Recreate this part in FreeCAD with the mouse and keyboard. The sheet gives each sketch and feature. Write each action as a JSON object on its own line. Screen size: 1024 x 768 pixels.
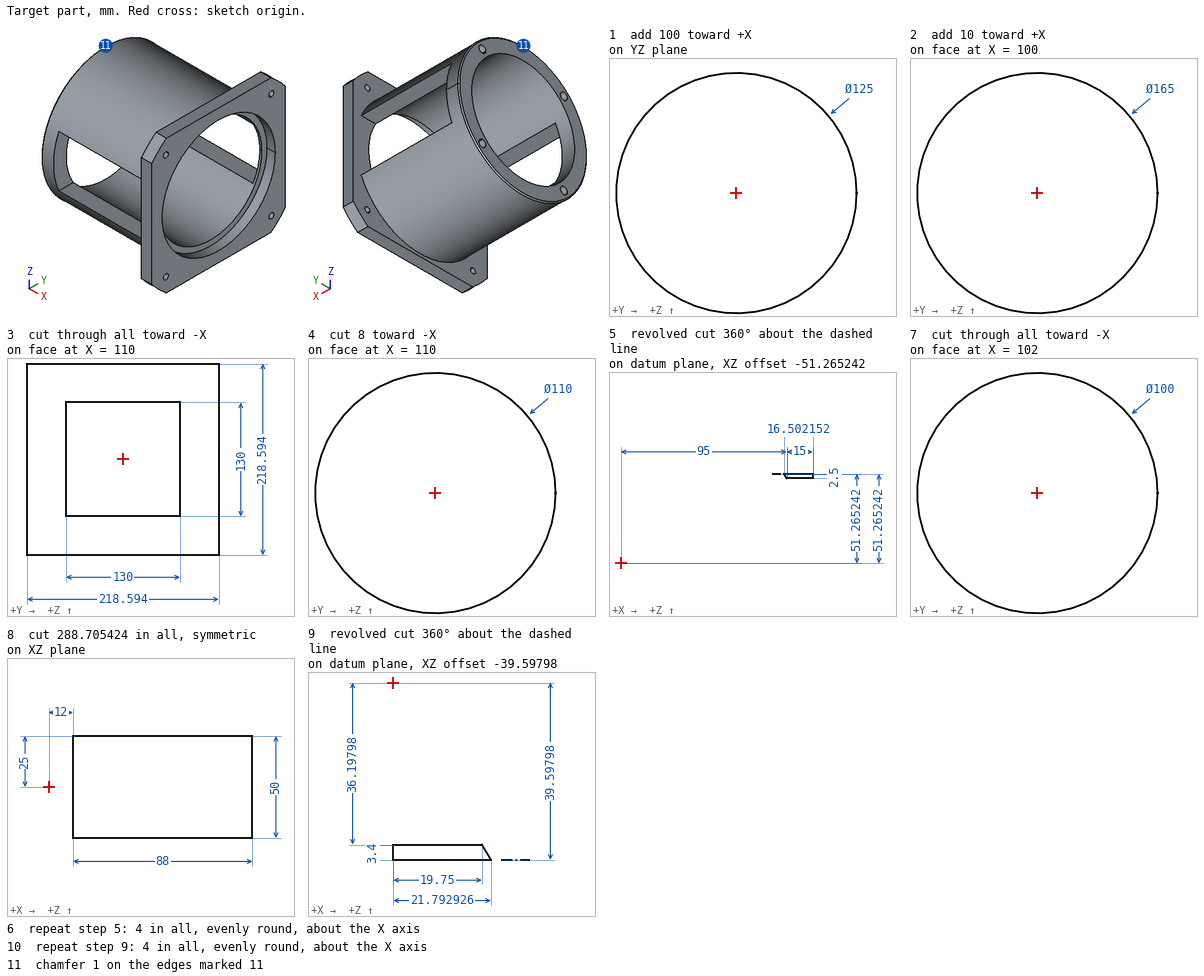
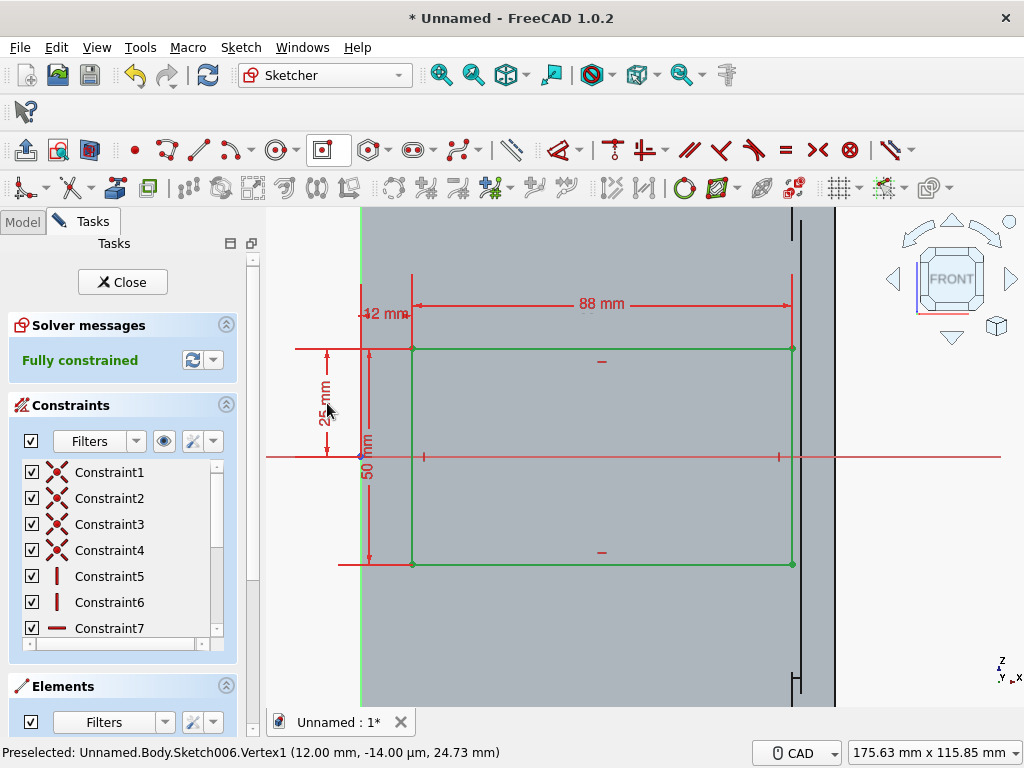
{"action": "left_click", "coordinate": [123, 282]}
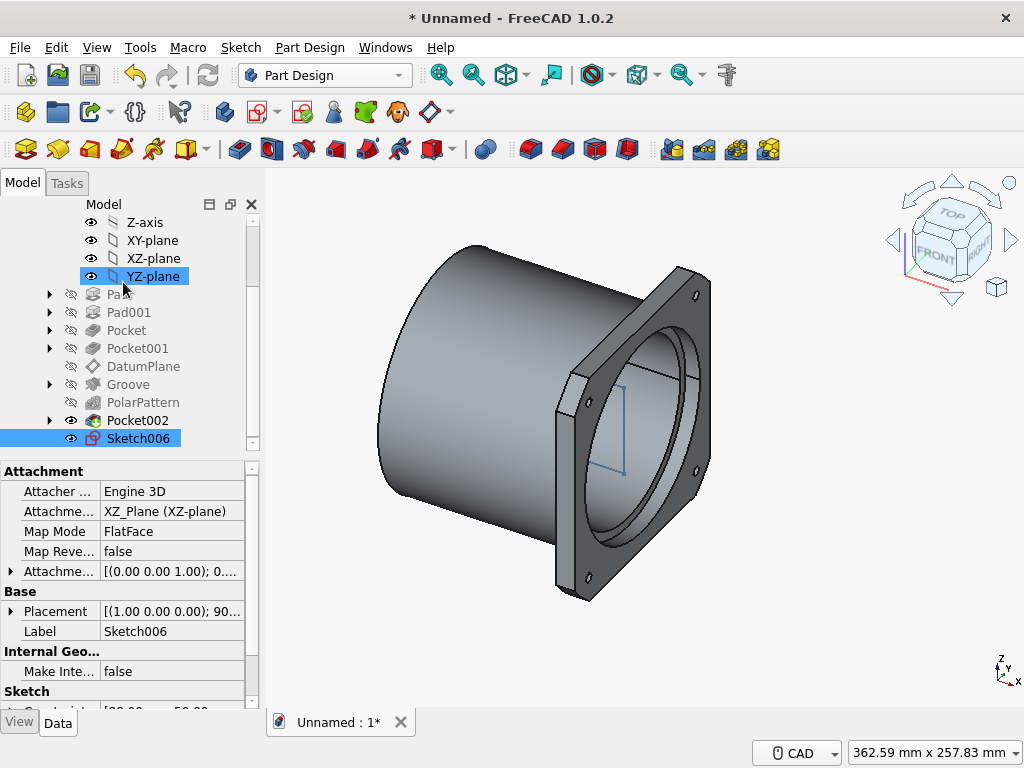
{"action": "left_click", "coordinate": [240, 150]}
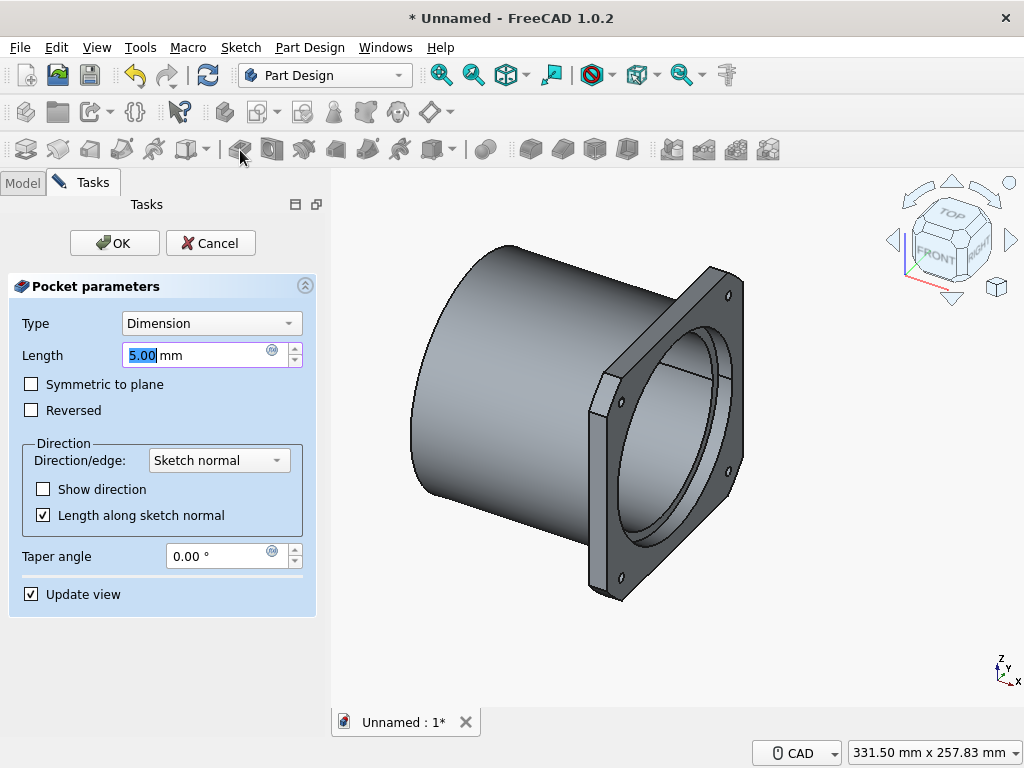
{"action": "type", "text": "288.705424"}
{"action": "key", "text": "Tab"}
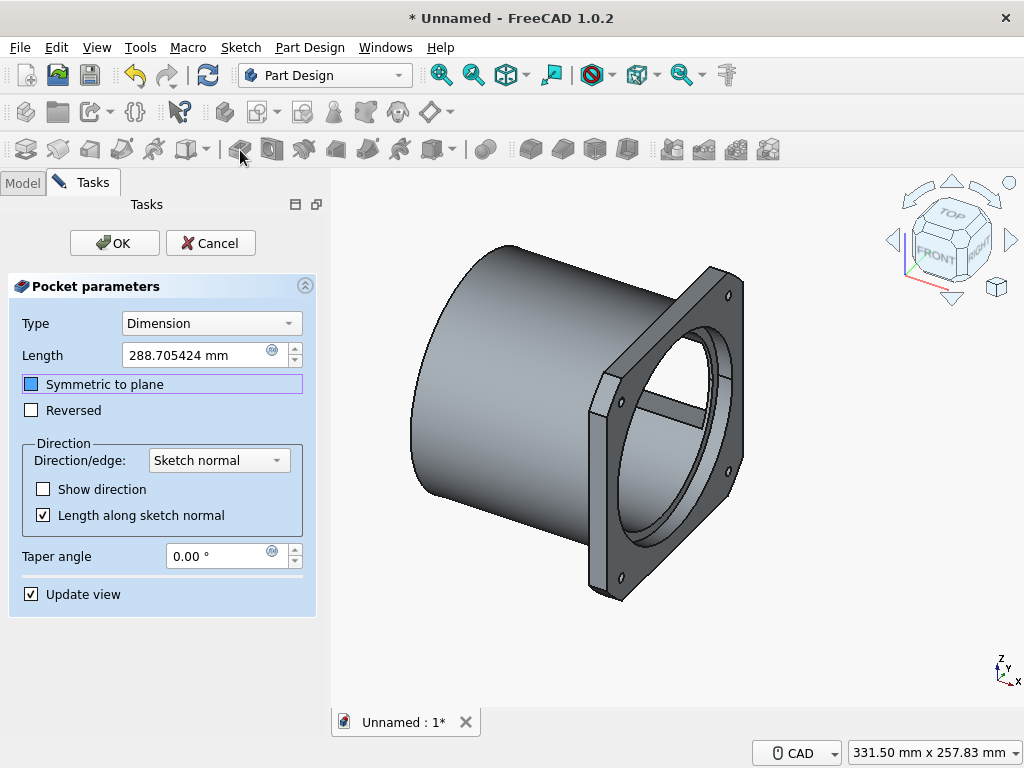
{"action": "left_click", "coordinate": [30, 384]}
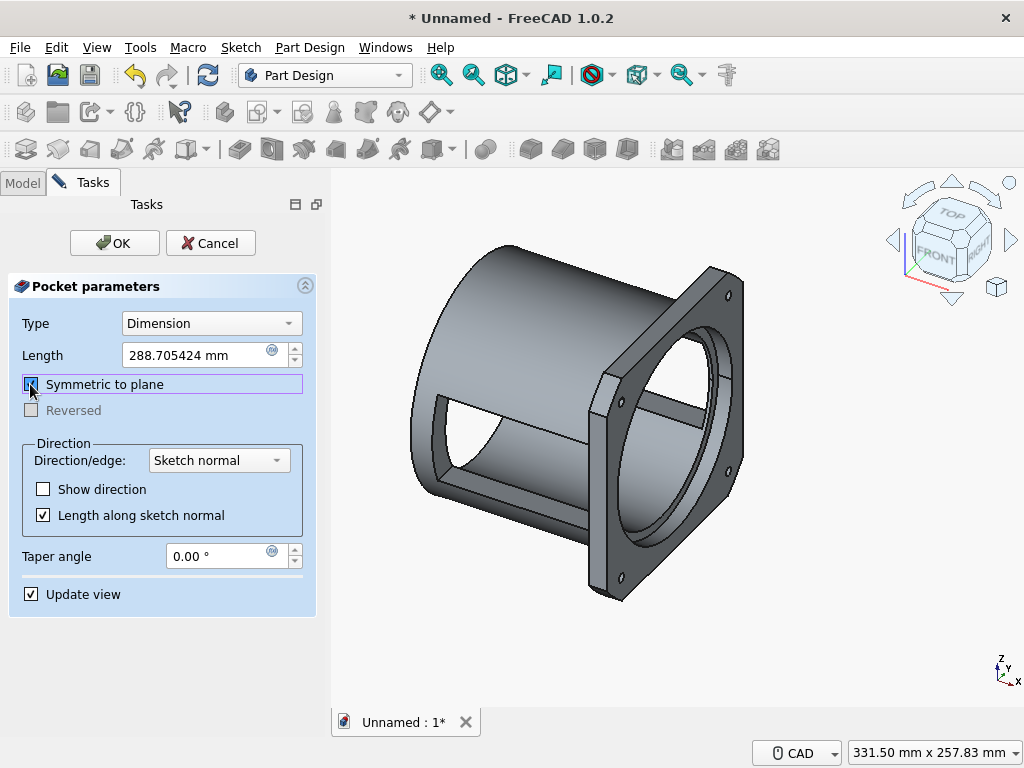
{"action": "left_click", "coordinate": [115, 243]}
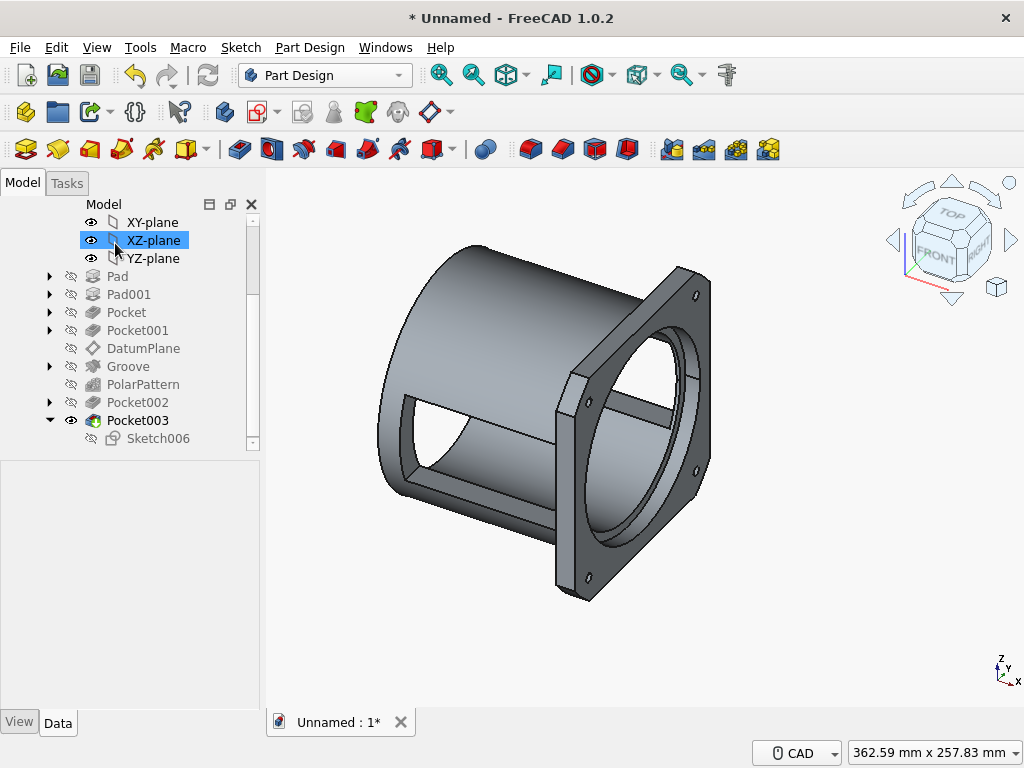
{"action": "scroll", "coordinate": [160, 326], "scroll_direction": "down", "scroll_amount": 3}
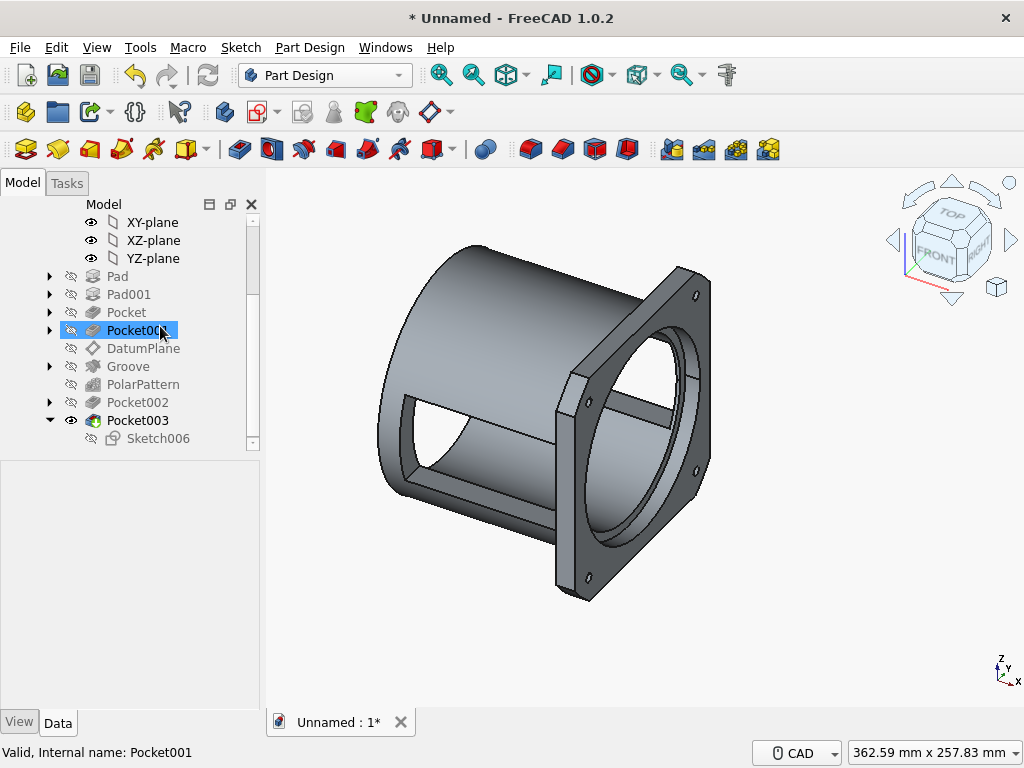
{"action": "scroll", "coordinate": [160, 326], "scroll_direction": "up", "scroll_amount": 15}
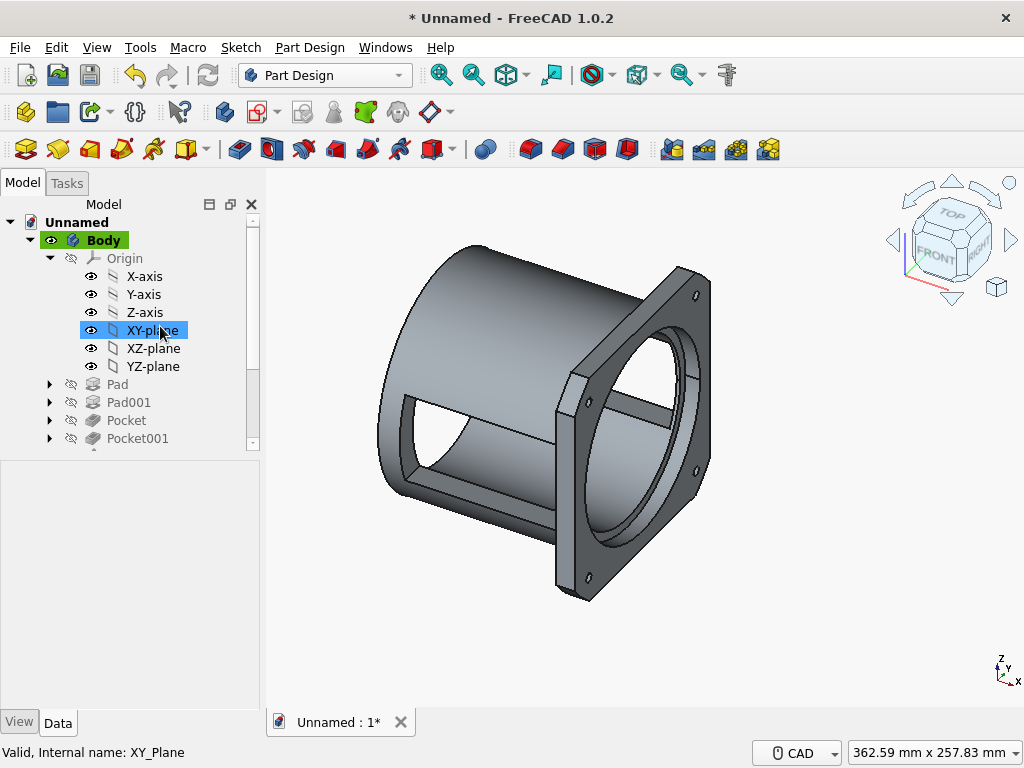
{"action": "left_click", "coordinate": [136, 348]}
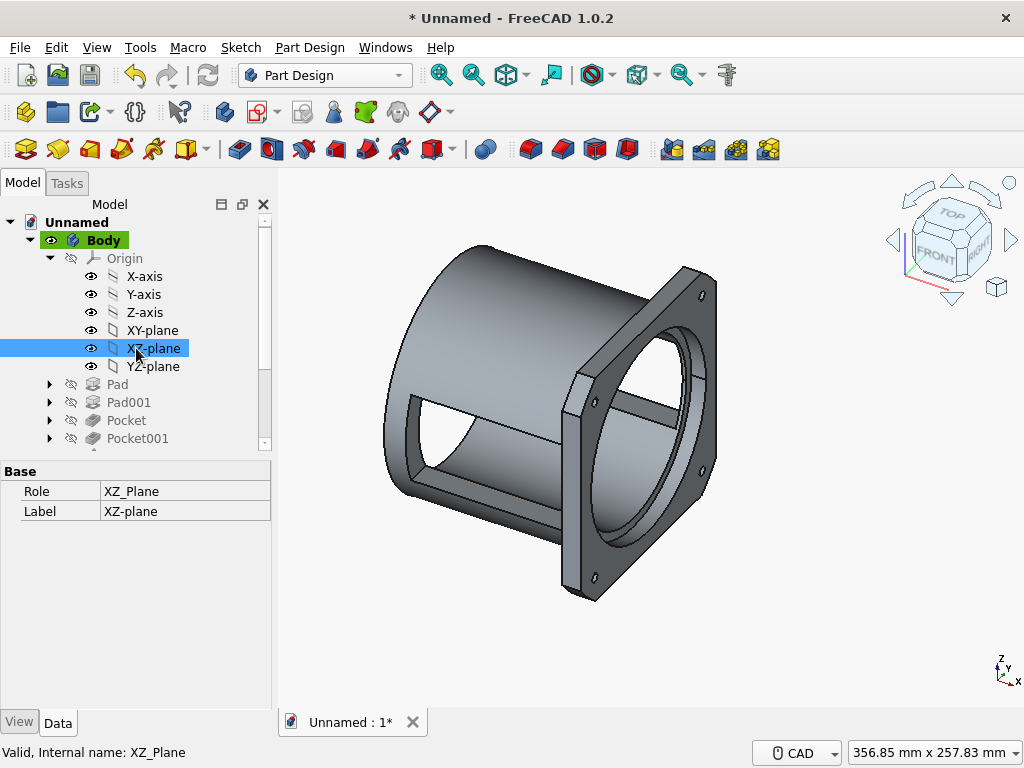
{"action": "left_click", "coordinate": [430, 112]}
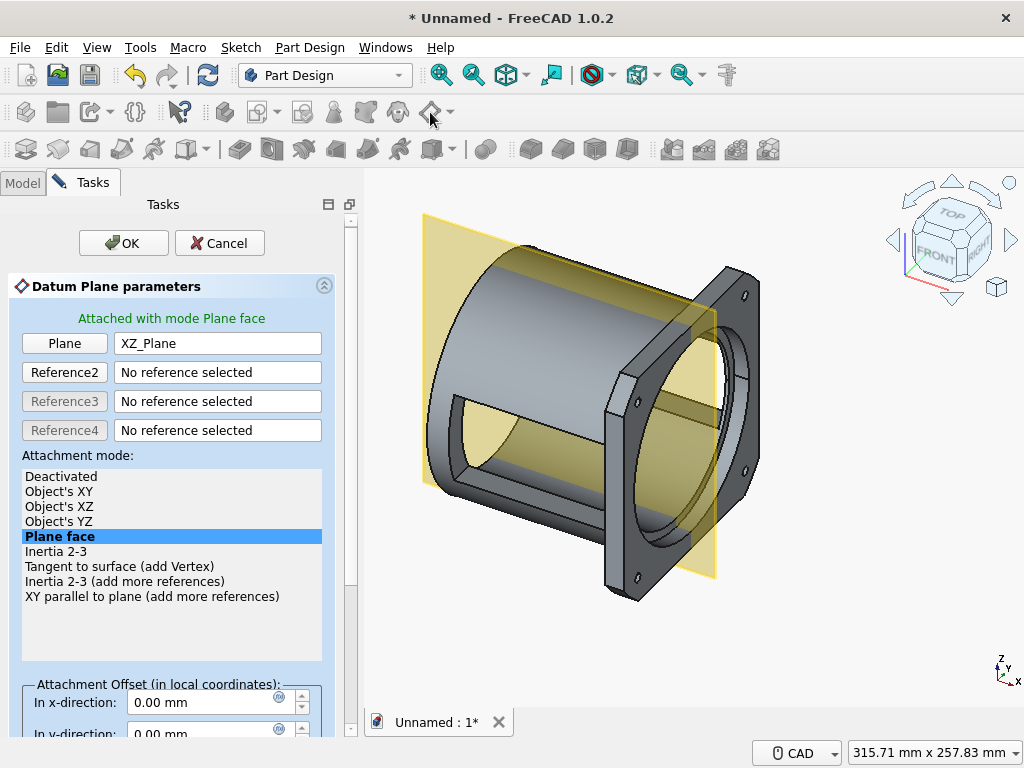
{"action": "scroll", "coordinate": [351, 475], "scroll_direction": "down", "scroll_amount": 2}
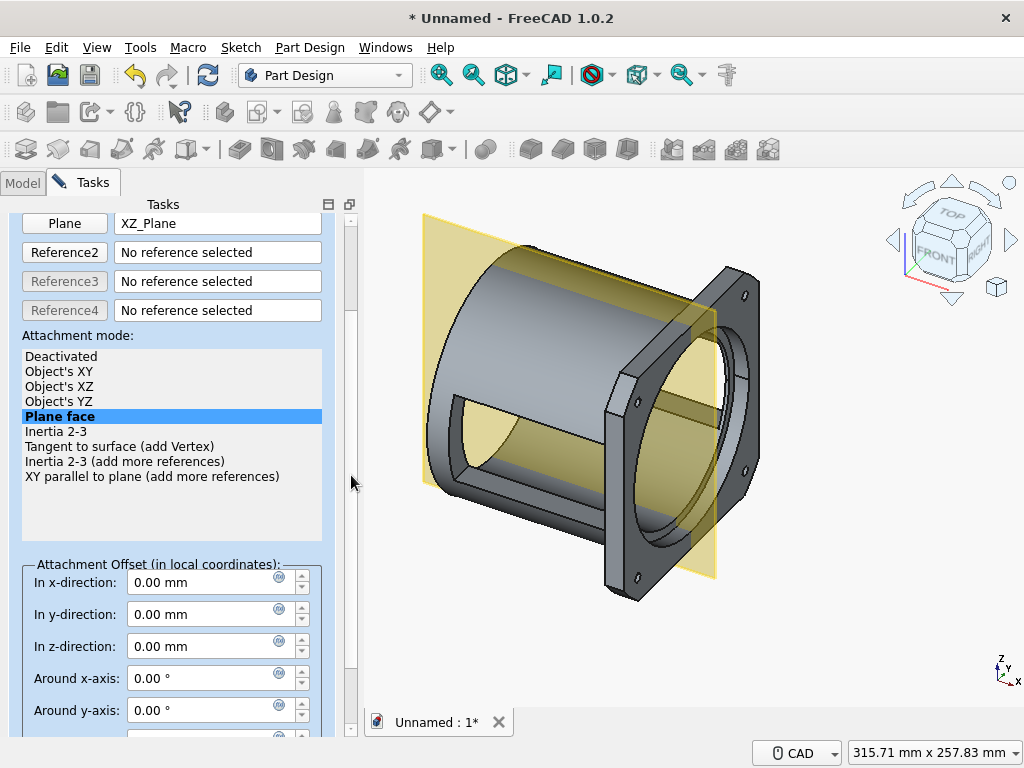
{"action": "triple_click", "coordinate": [210, 646]}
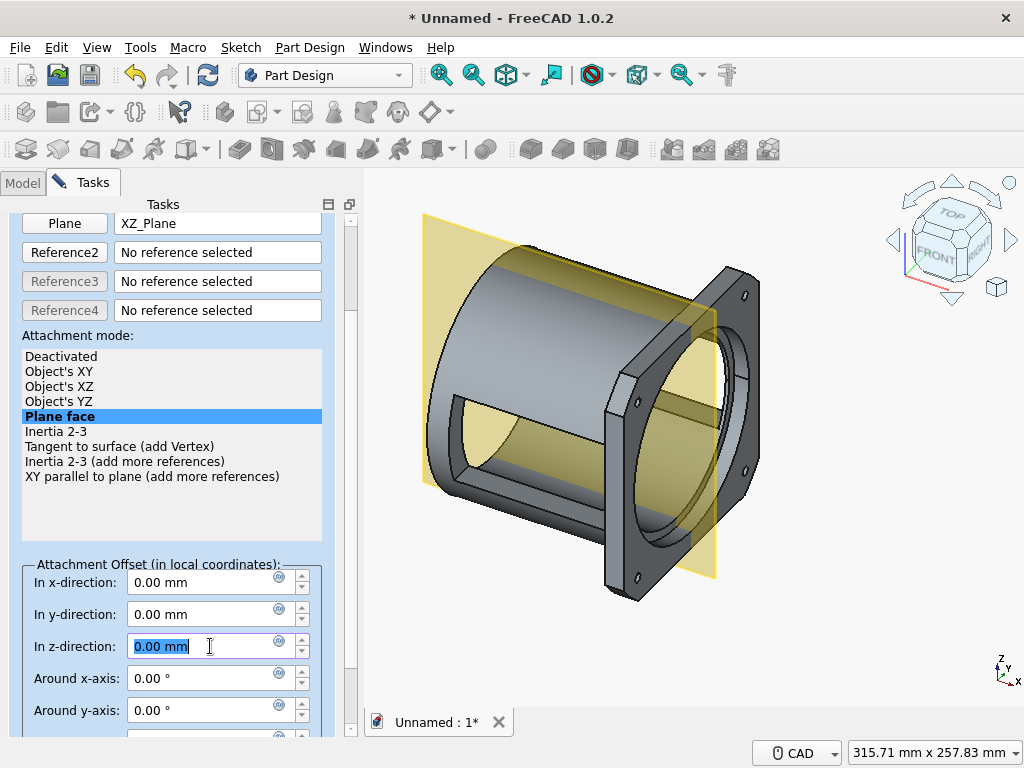
{"action": "type", "text": "-39.59798"}
{"action": "key", "text": "Tab"}